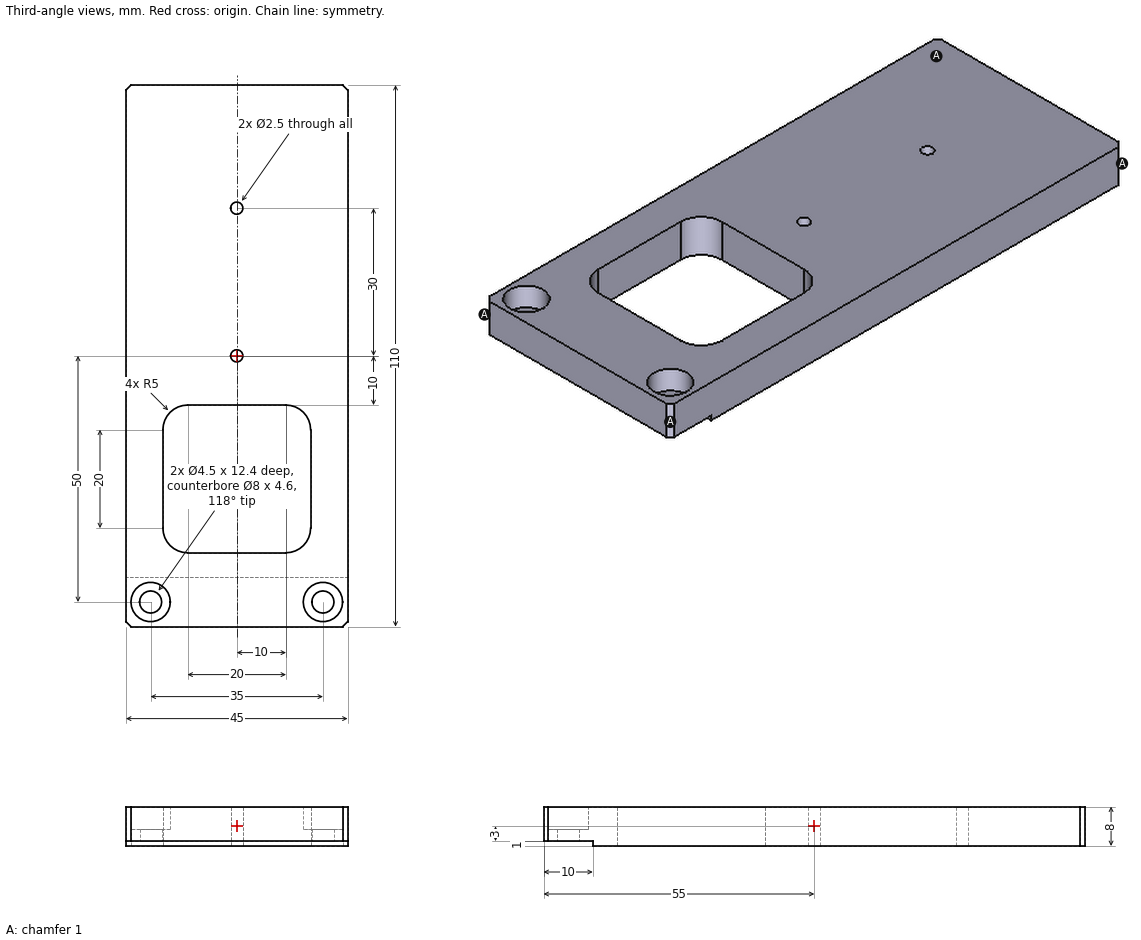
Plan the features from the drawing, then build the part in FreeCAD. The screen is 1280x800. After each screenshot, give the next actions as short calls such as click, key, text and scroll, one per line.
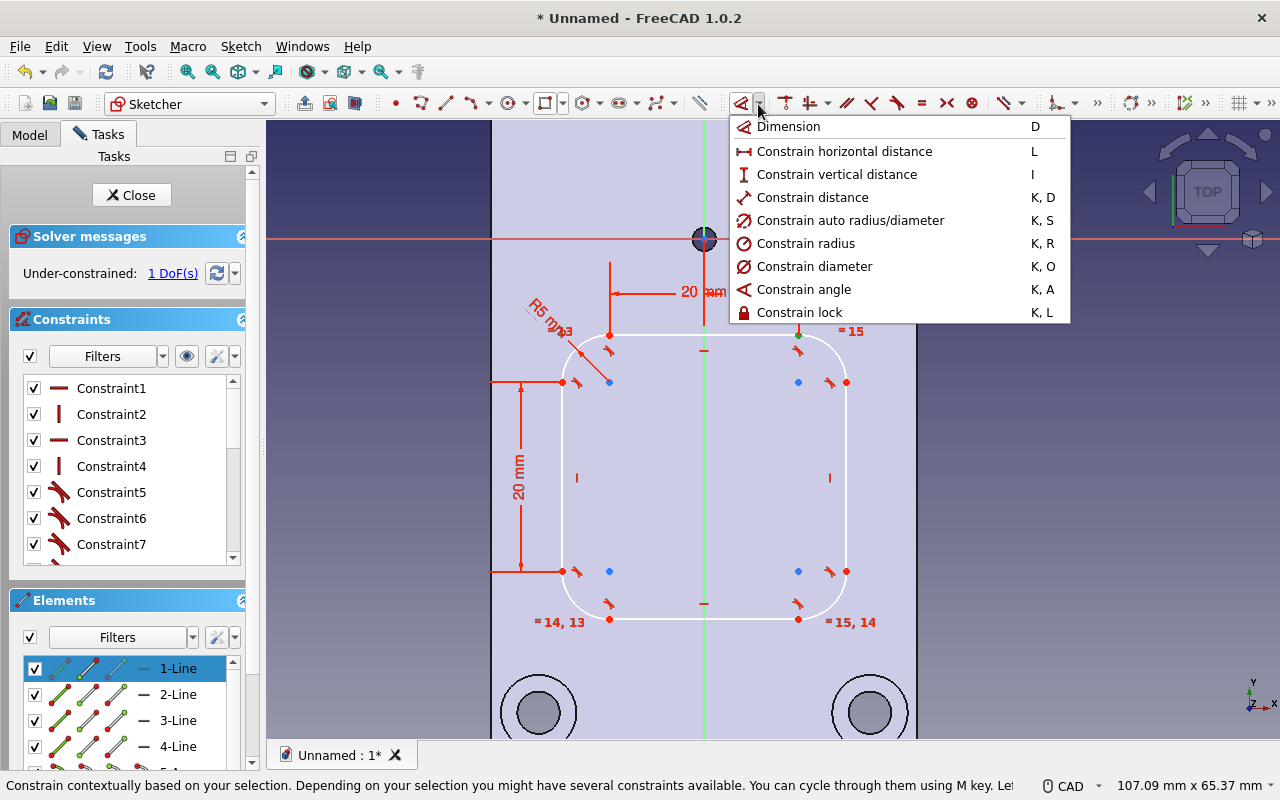
click(900, 174)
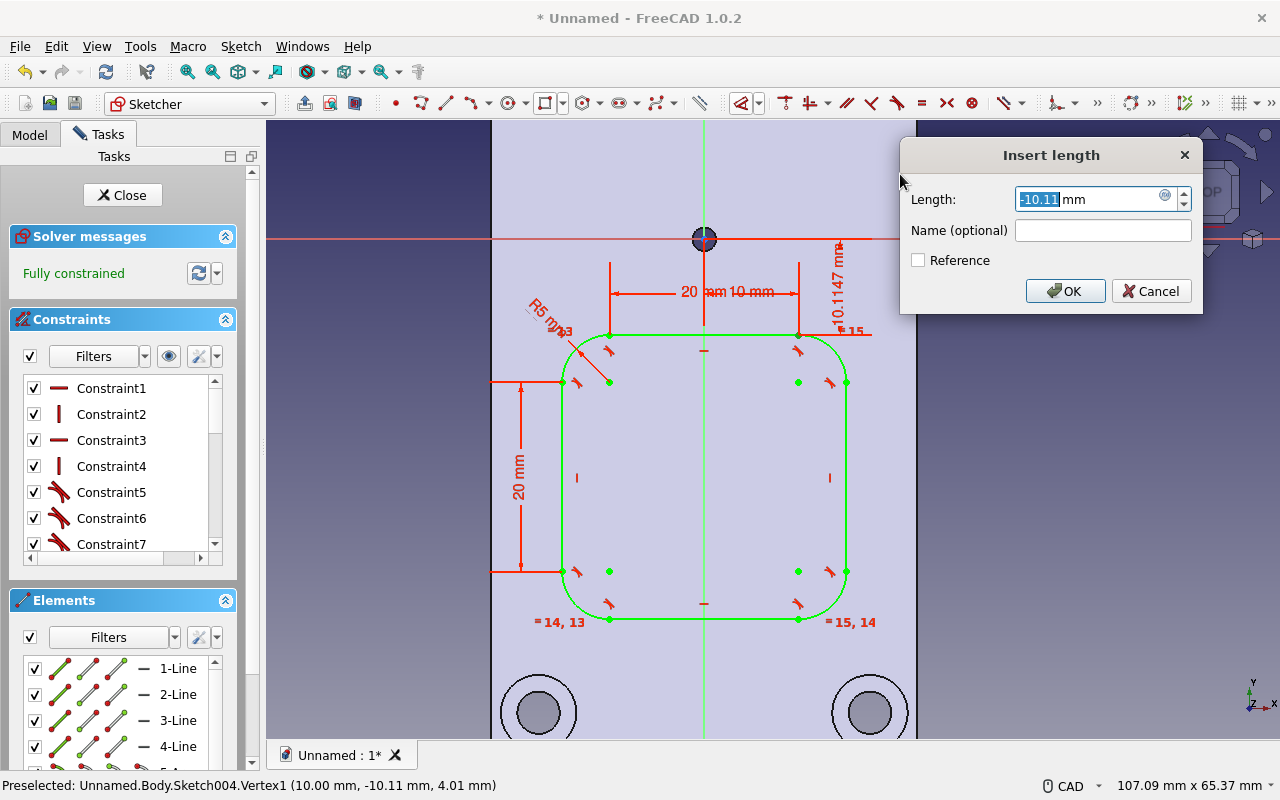
text(-10)
key(Return)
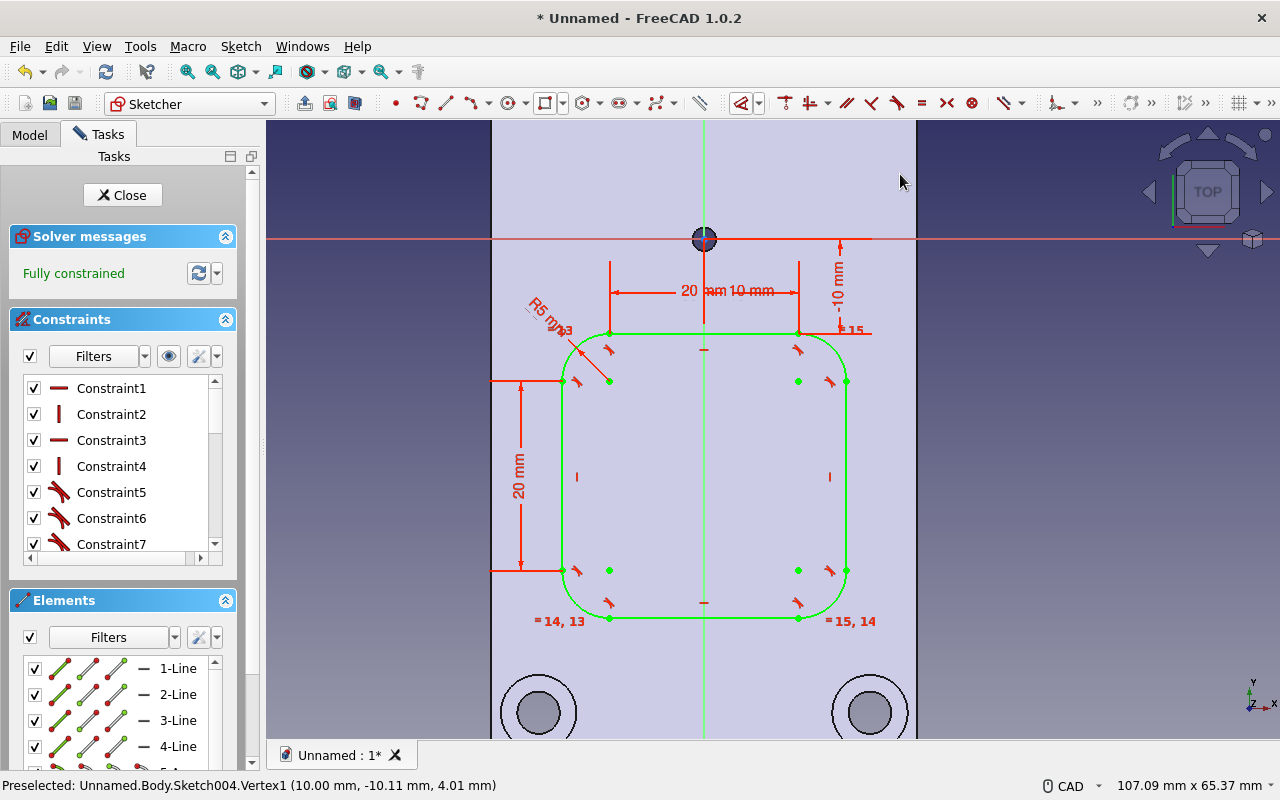
click(123, 195)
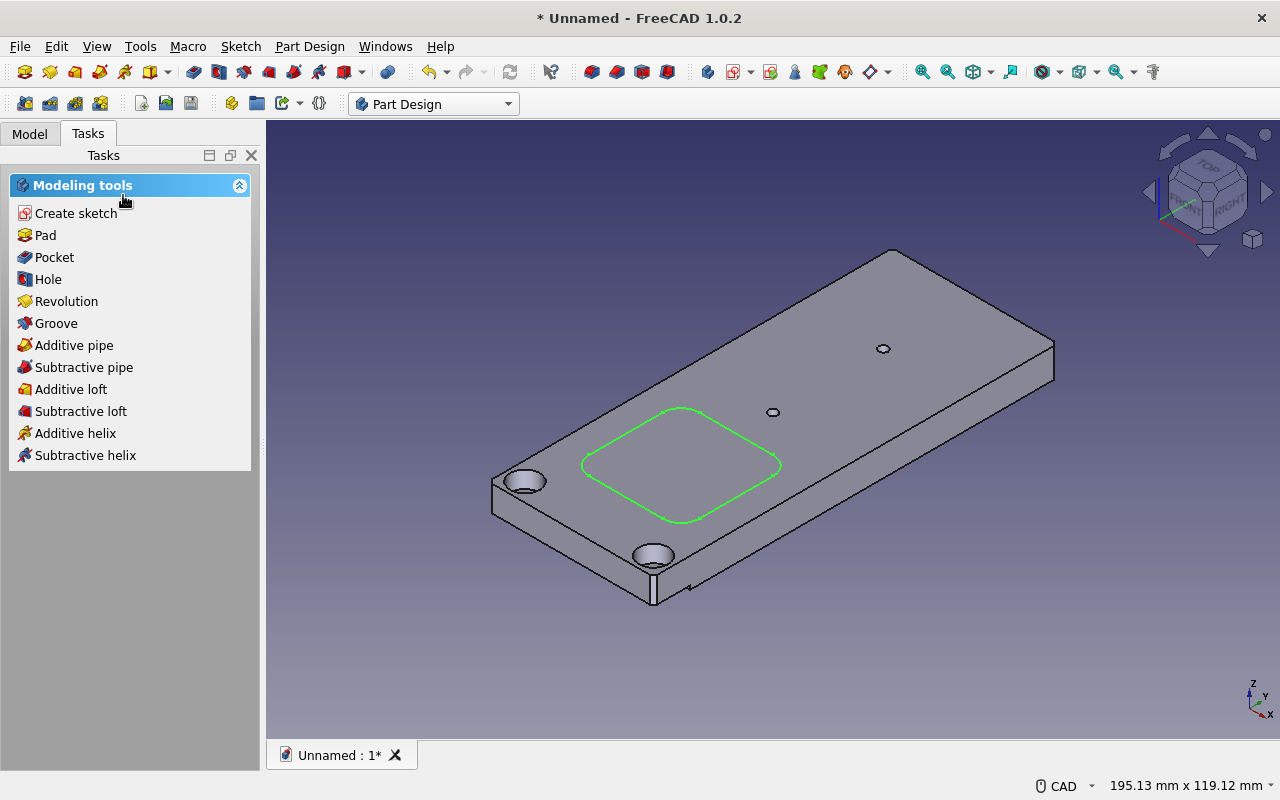
click(194, 72)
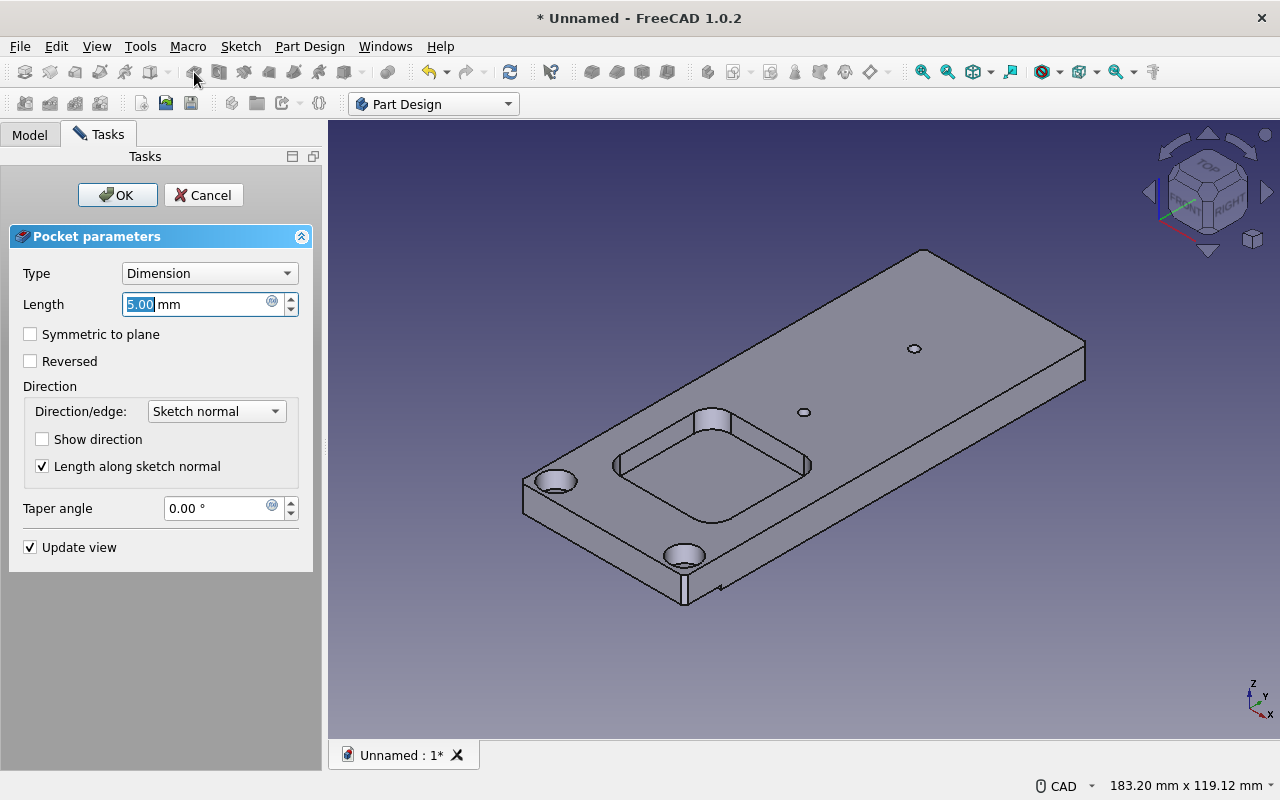
click(210, 274)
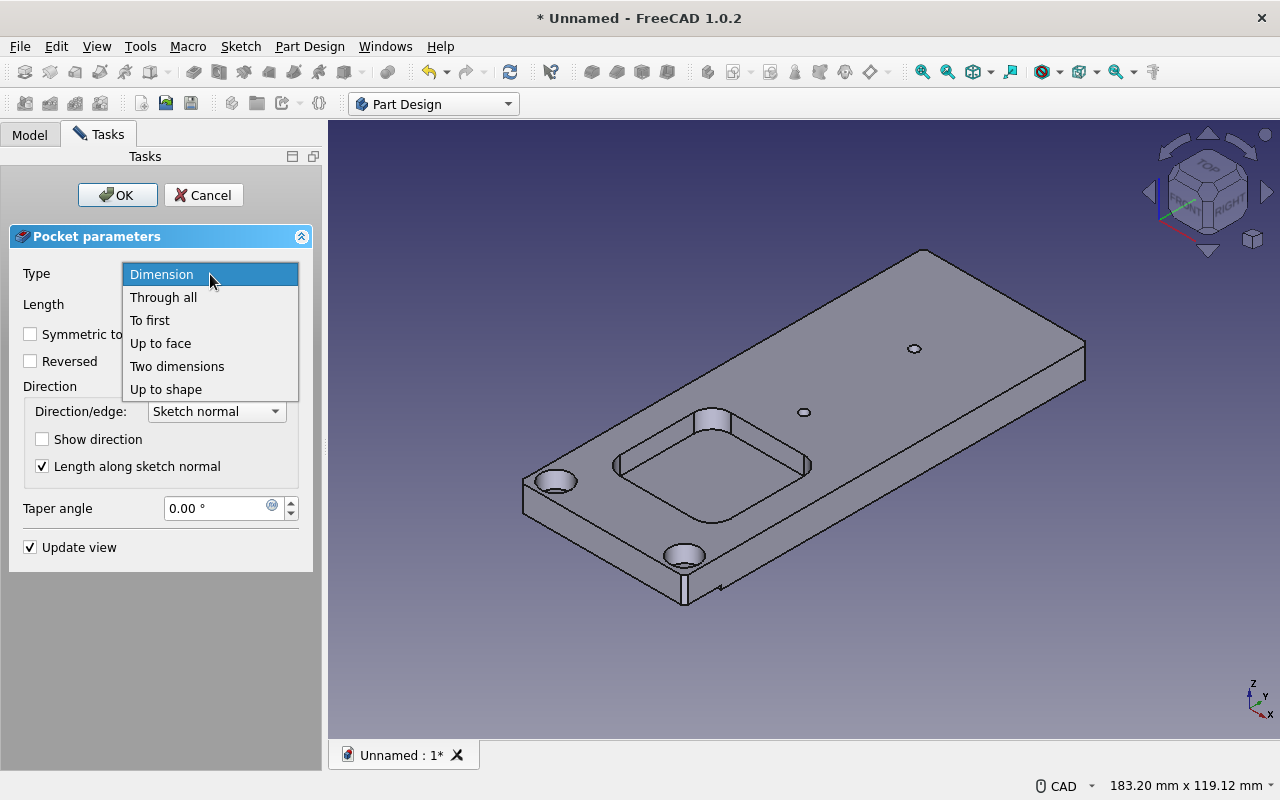
click(208, 298)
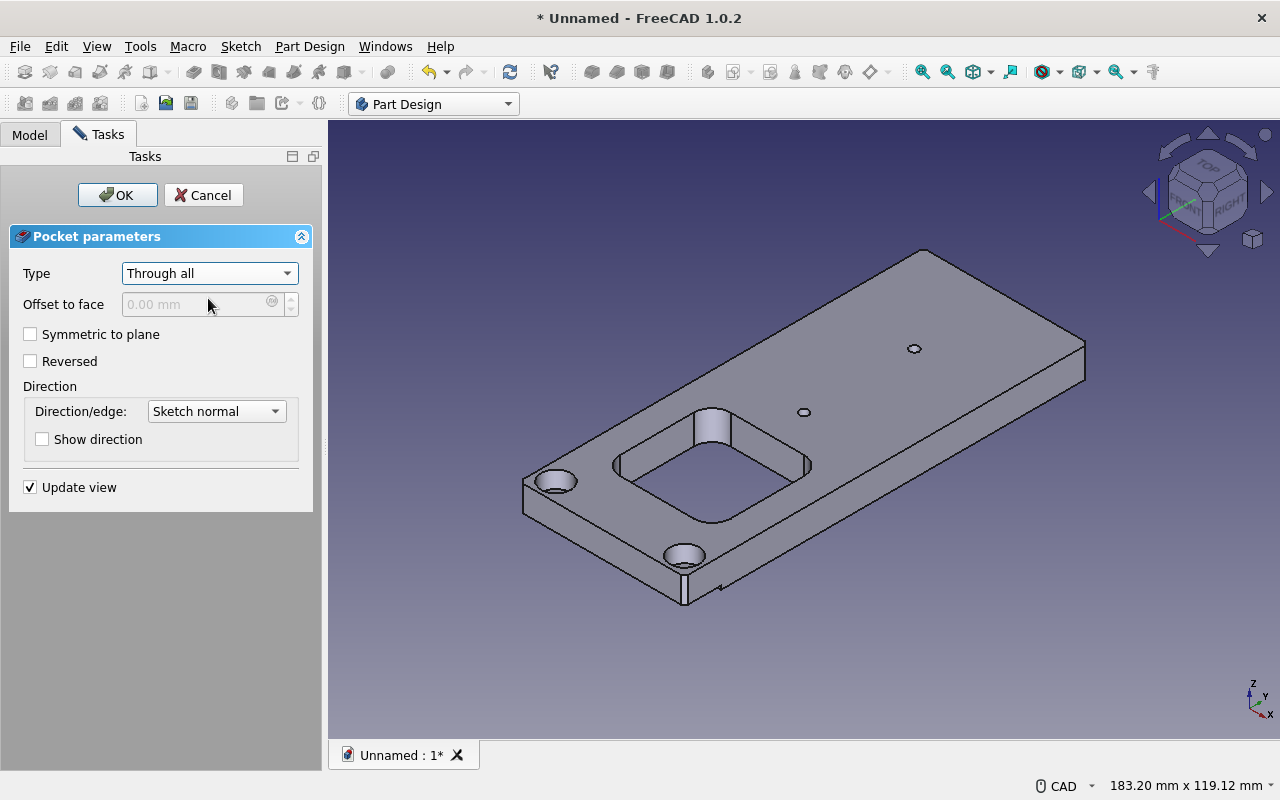
click(118, 195)